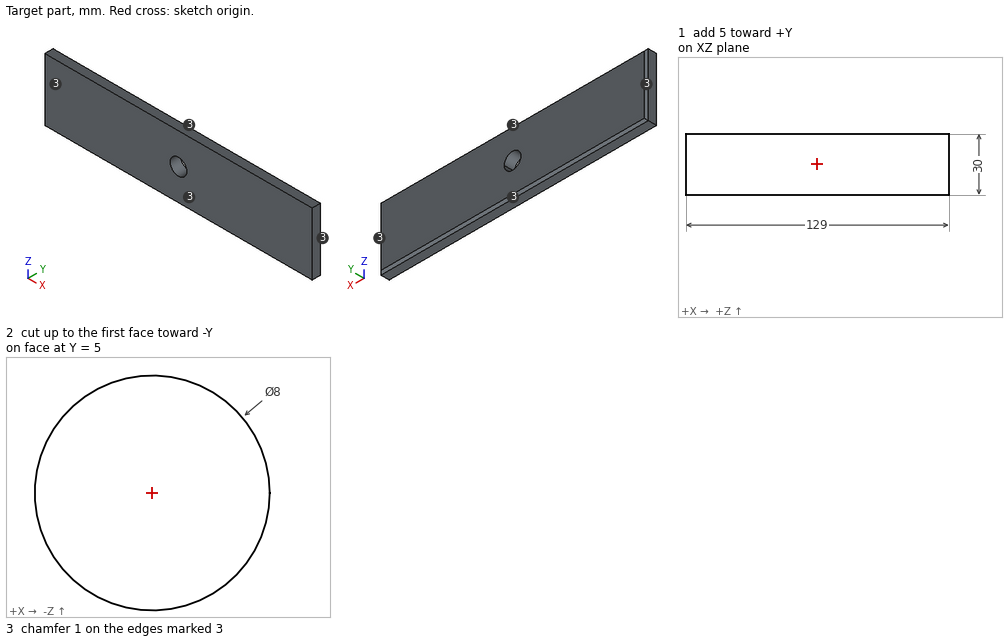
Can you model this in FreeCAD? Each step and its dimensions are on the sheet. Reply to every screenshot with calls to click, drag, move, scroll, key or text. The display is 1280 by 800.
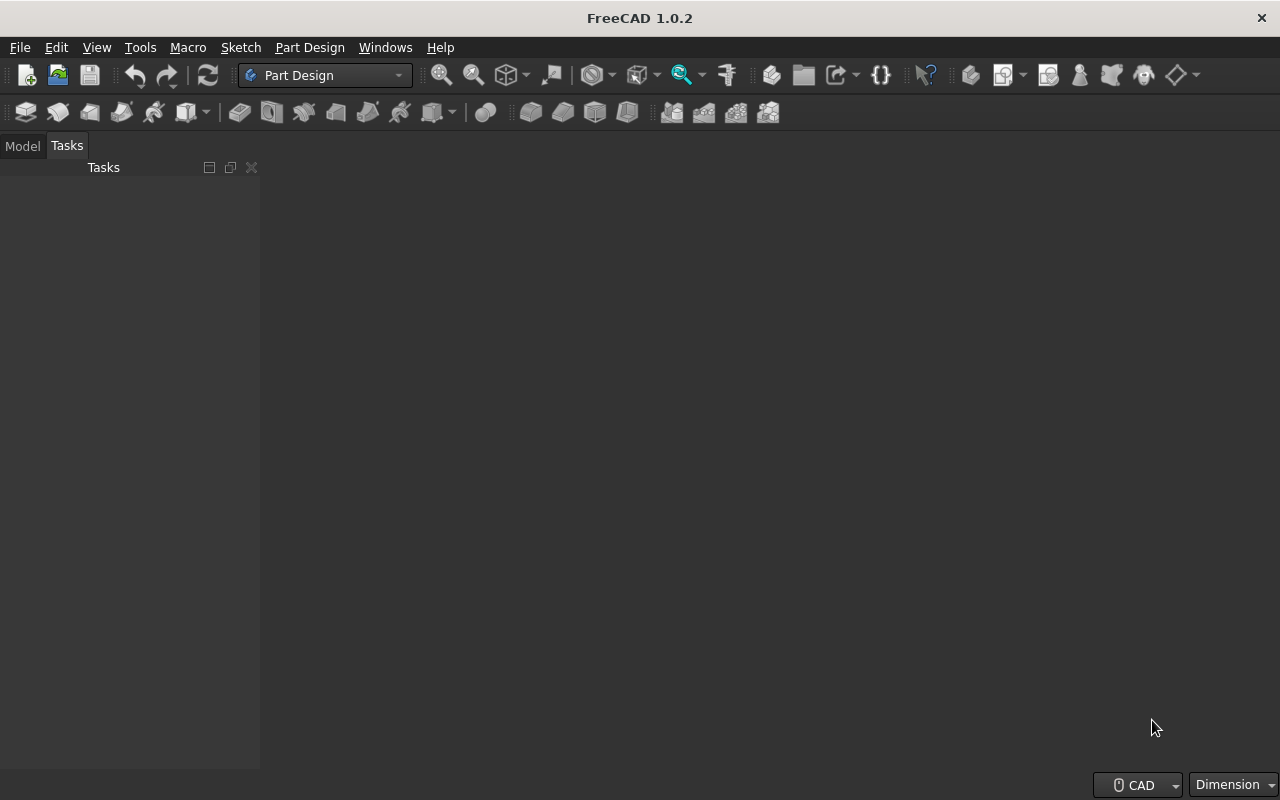
click(26, 76)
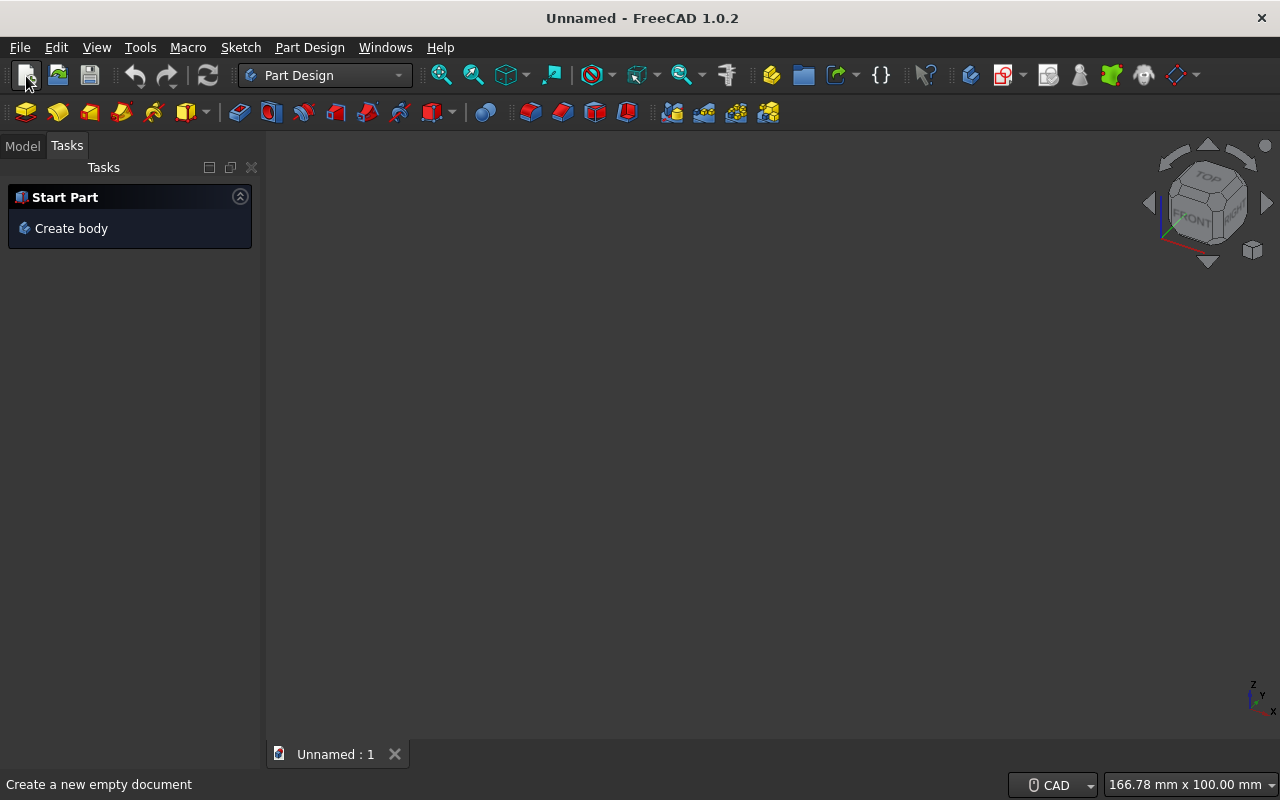
click(1004, 76)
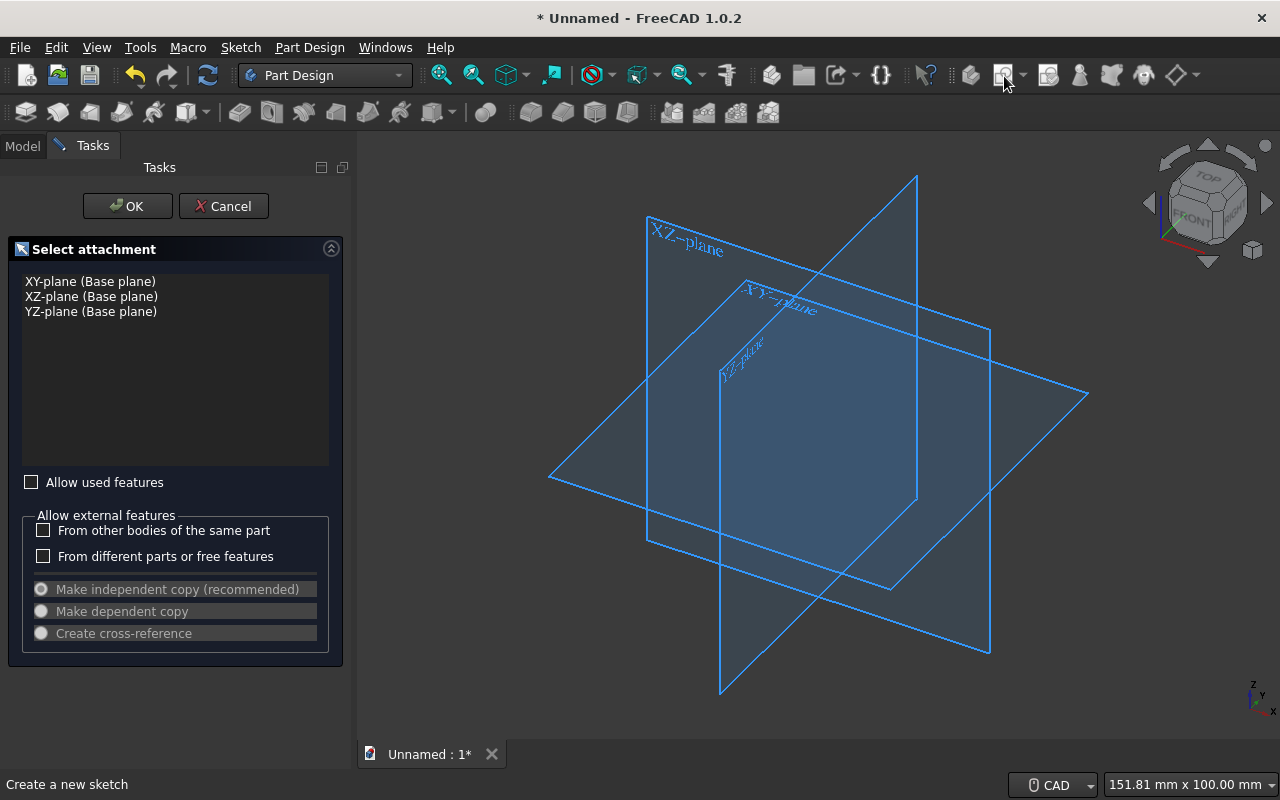
click(82, 296)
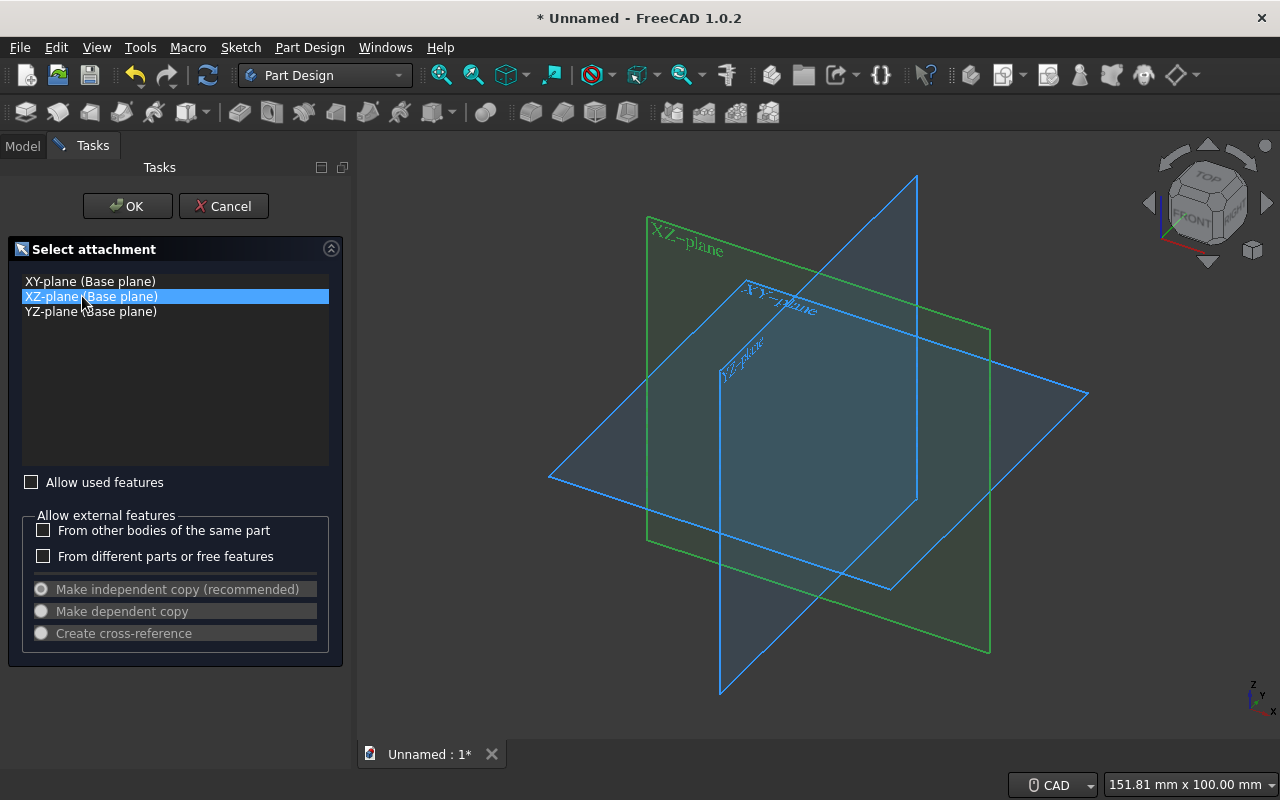
click(128, 206)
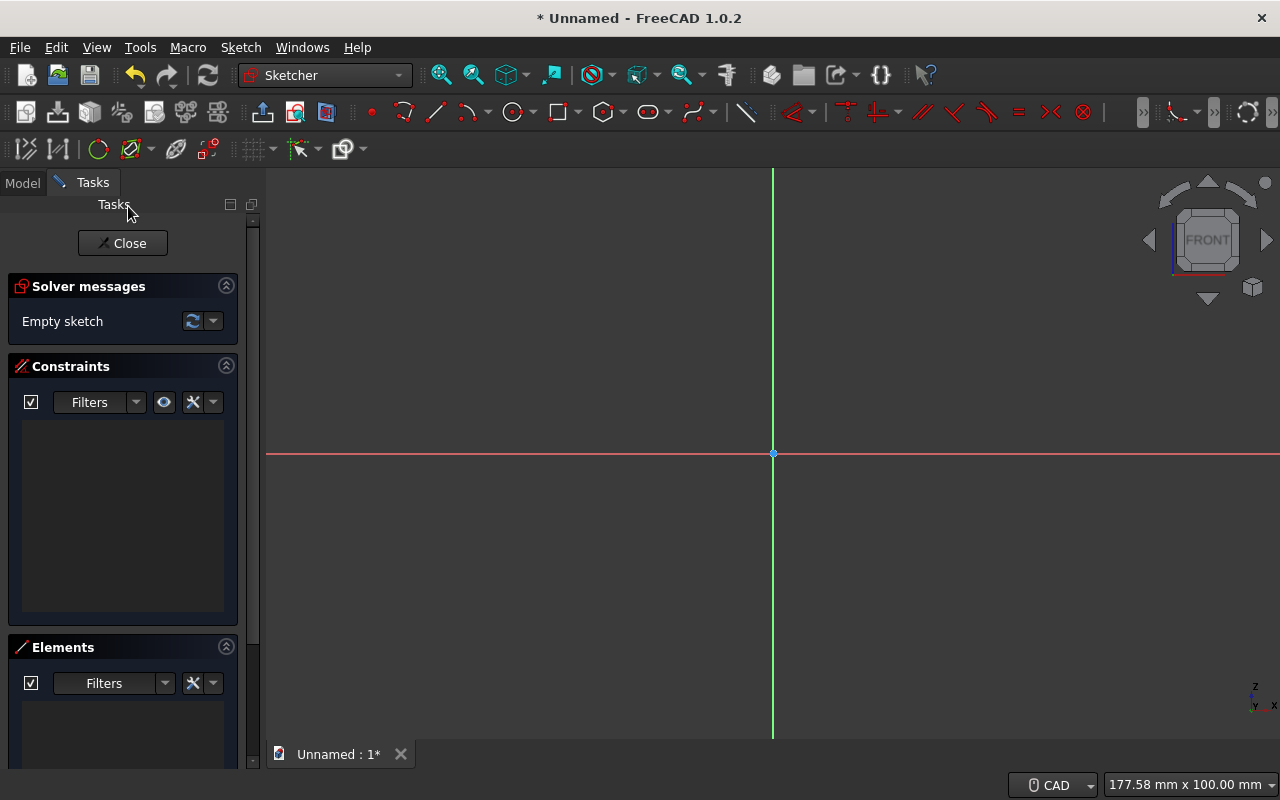
scroll(395, 453, down, 1)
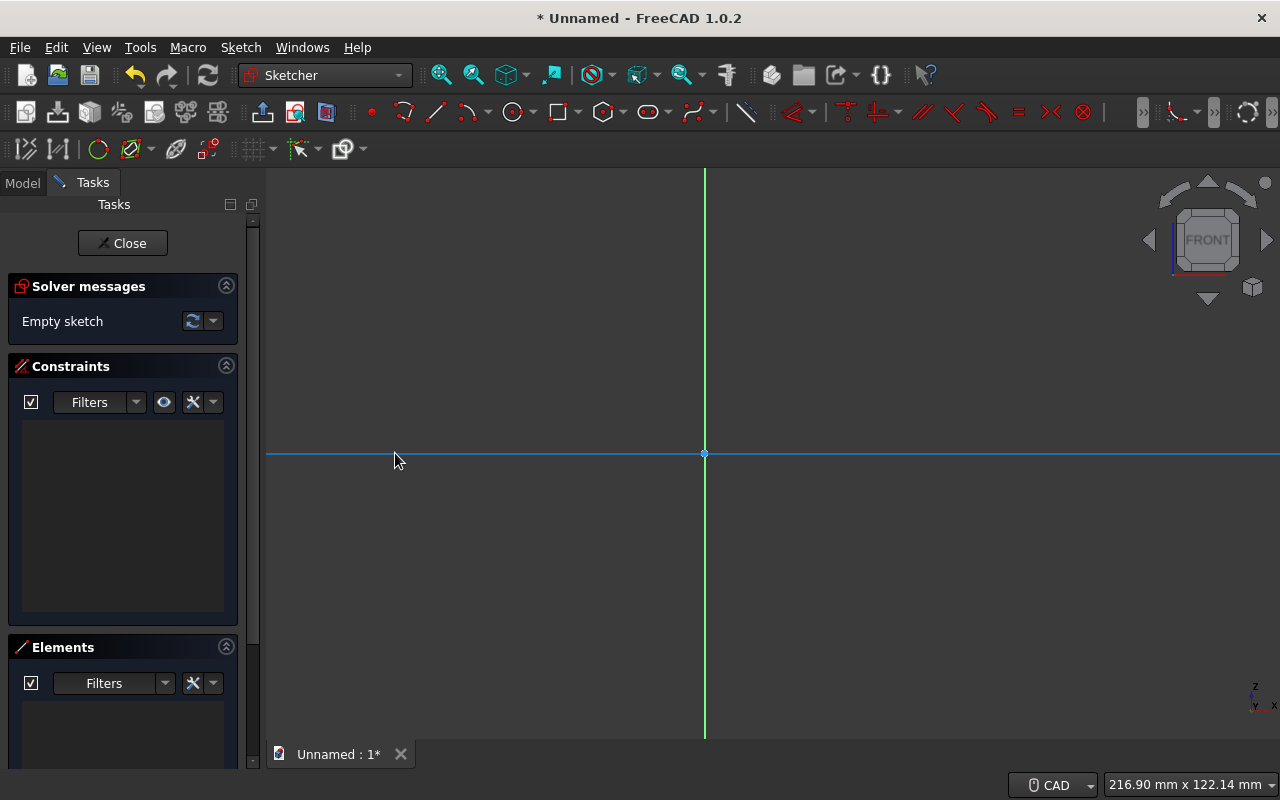
key(g)
key(v)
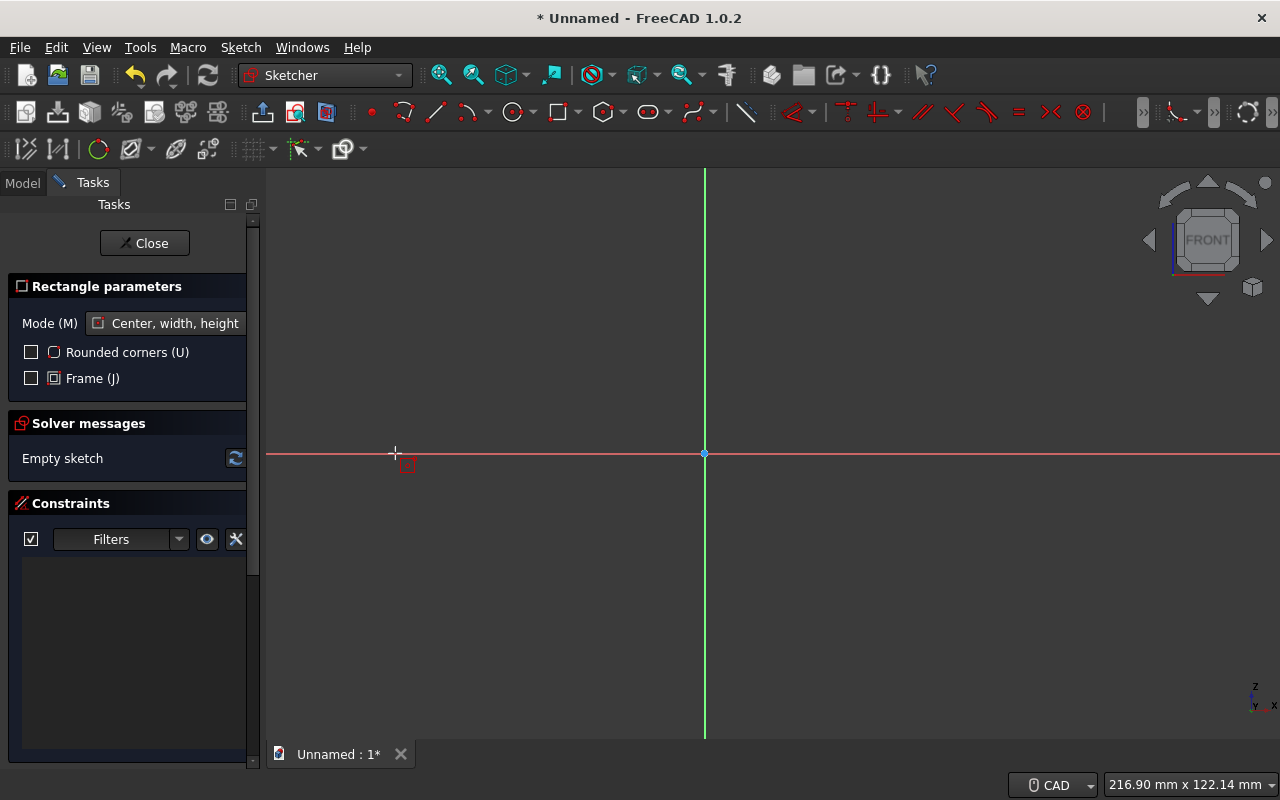
click(705, 454)
click(1006, 383)
key(Escape)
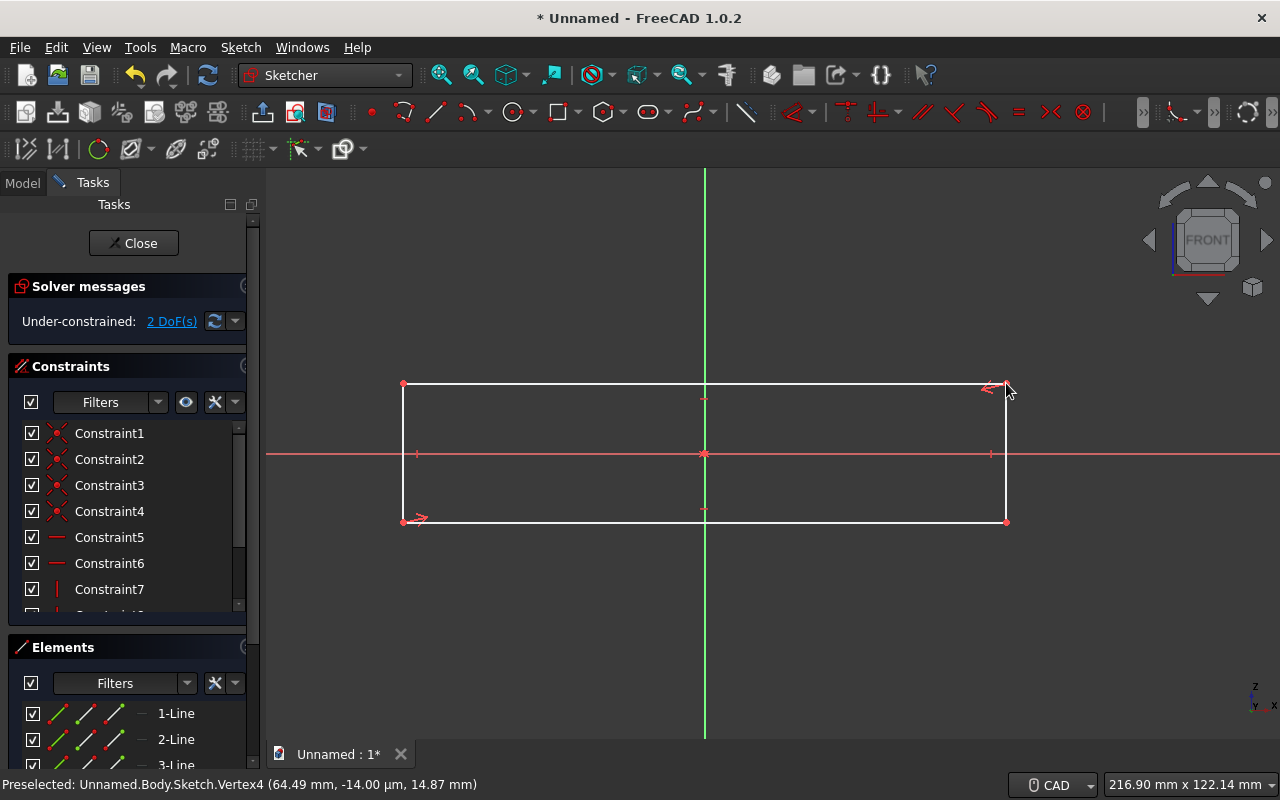
key(d)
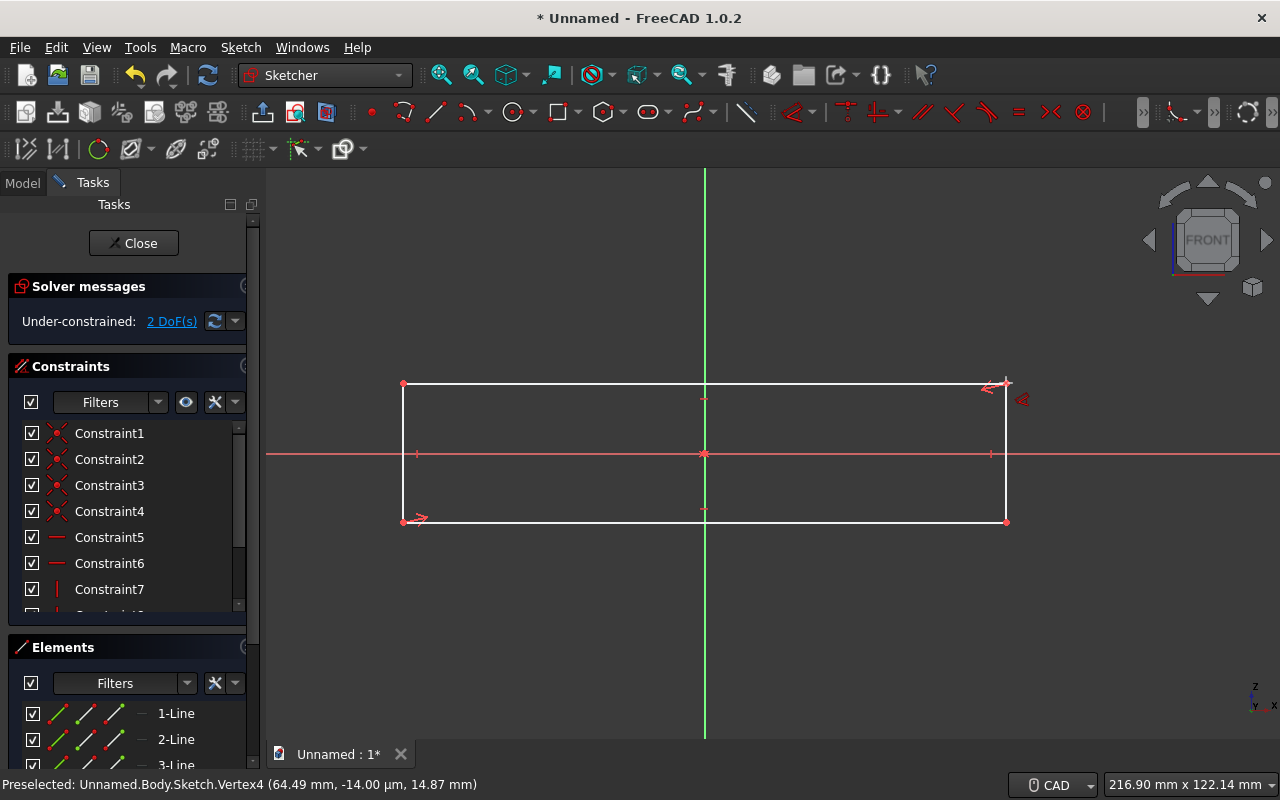
click(1006, 481)
click(1040, 422)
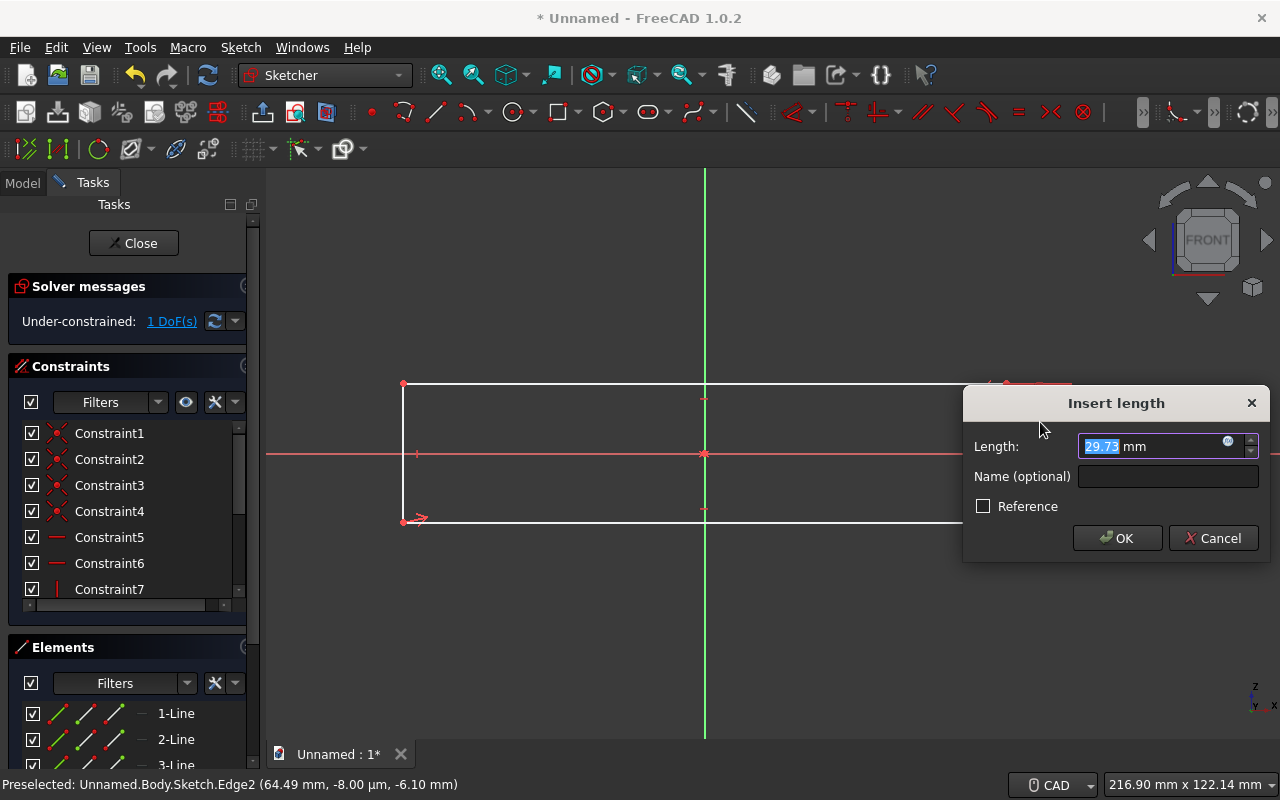
text(30)
key(Return)